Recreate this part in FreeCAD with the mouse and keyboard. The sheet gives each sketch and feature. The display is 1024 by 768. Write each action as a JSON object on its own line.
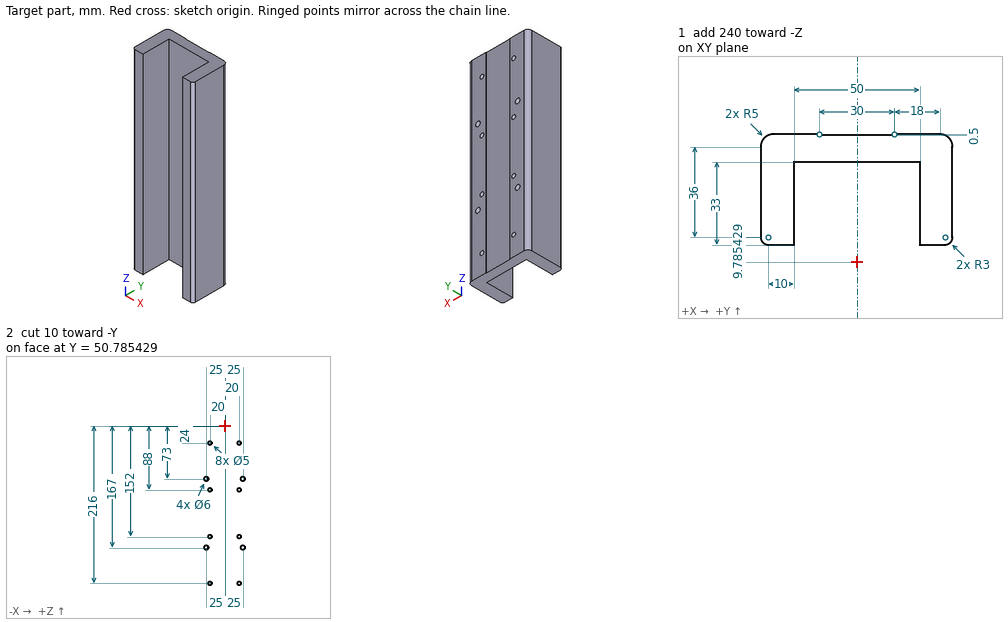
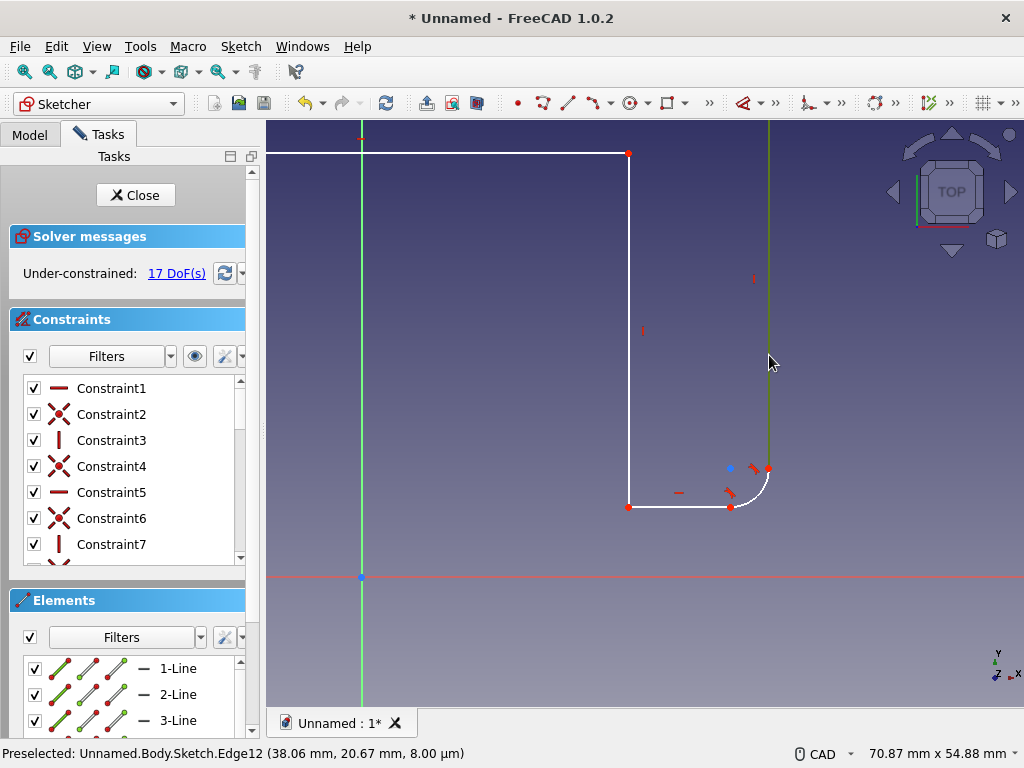
{"action": "scroll", "coordinate": [752, 502], "scroll_direction": "down", "scroll_amount": 4}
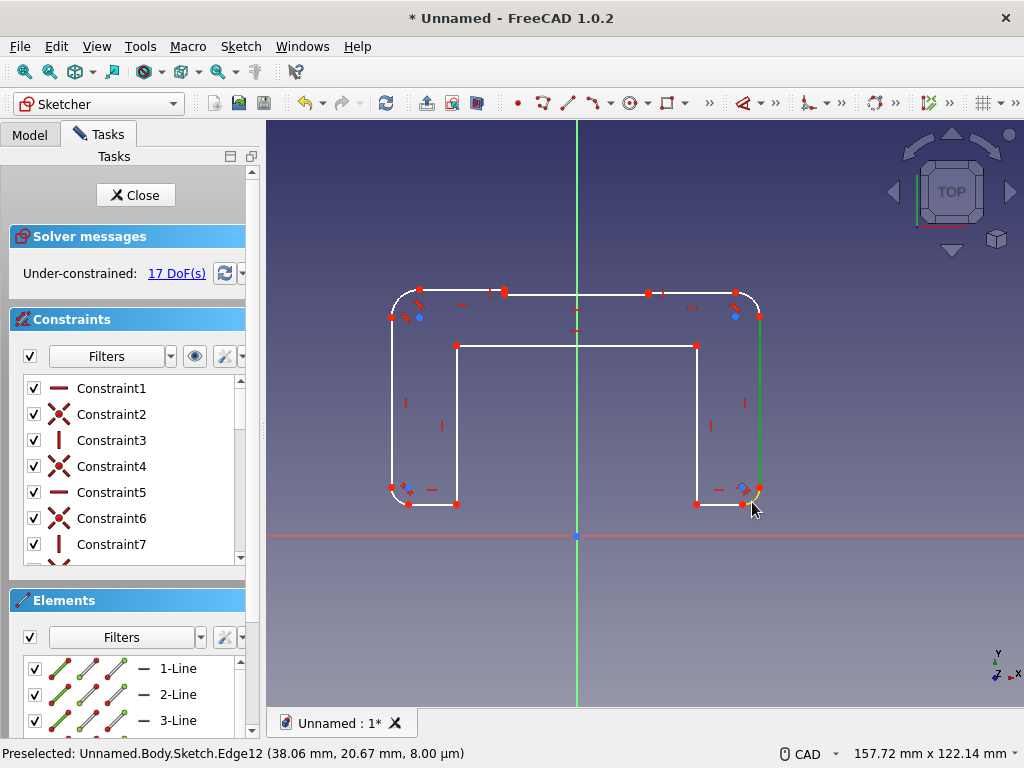
{"action": "scroll", "coordinate": [757, 306], "scroll_direction": "up", "scroll_amount": 2}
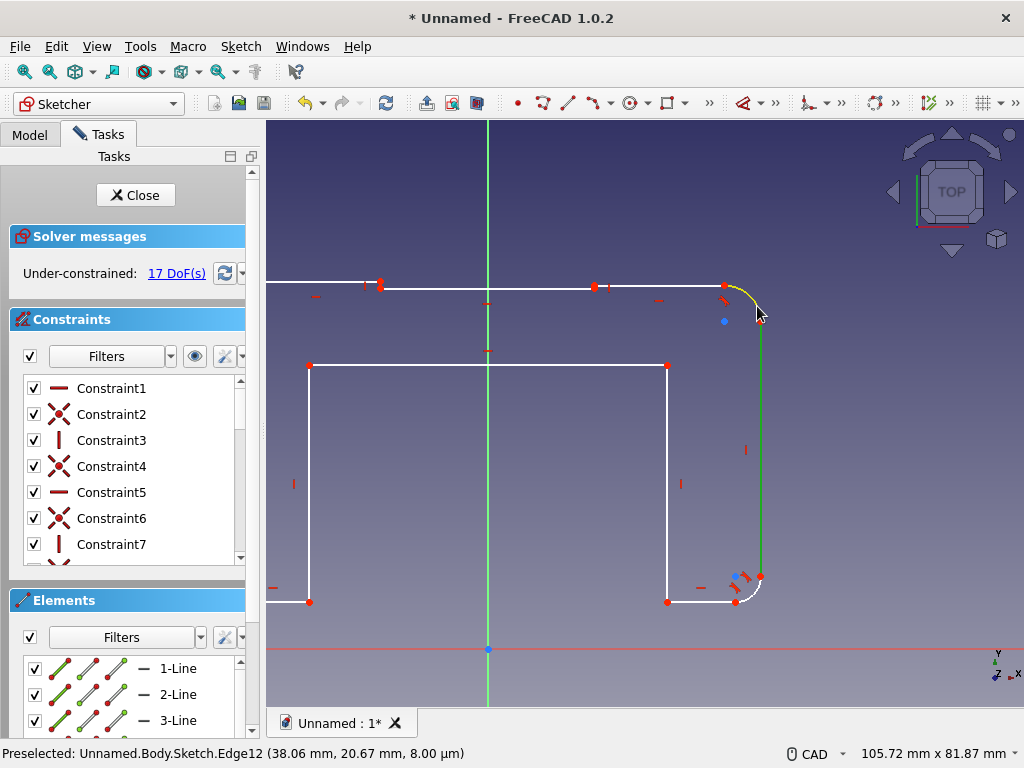
{"action": "left_click", "coordinate": [757, 305]}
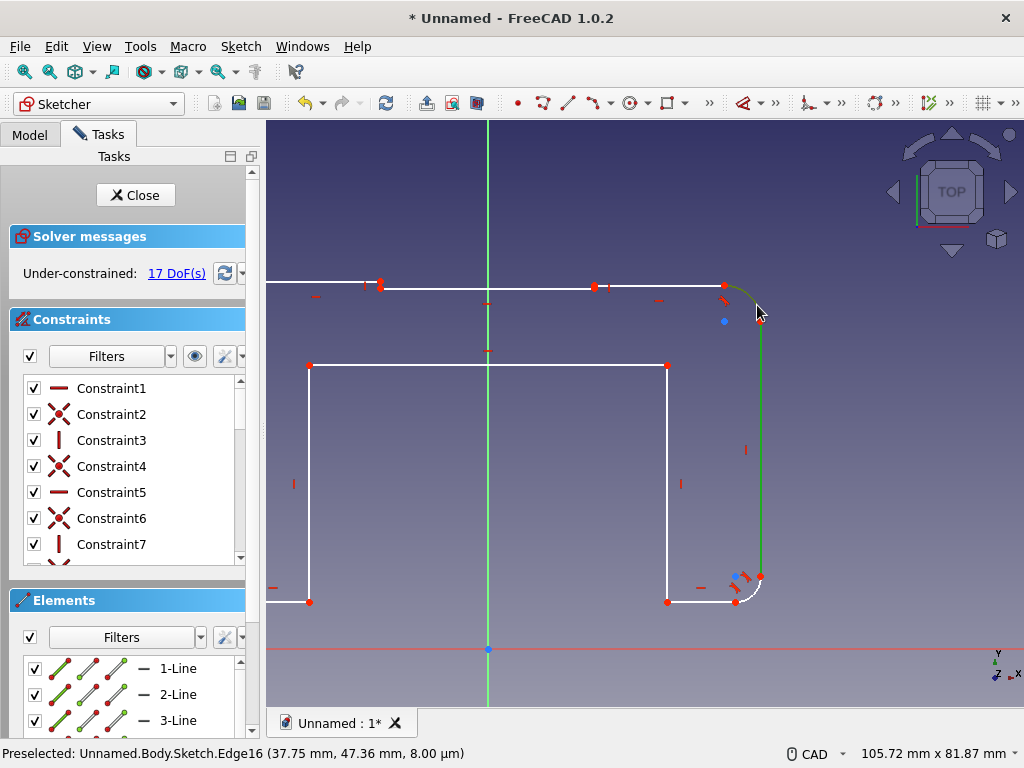
{"action": "key", "text": "t"}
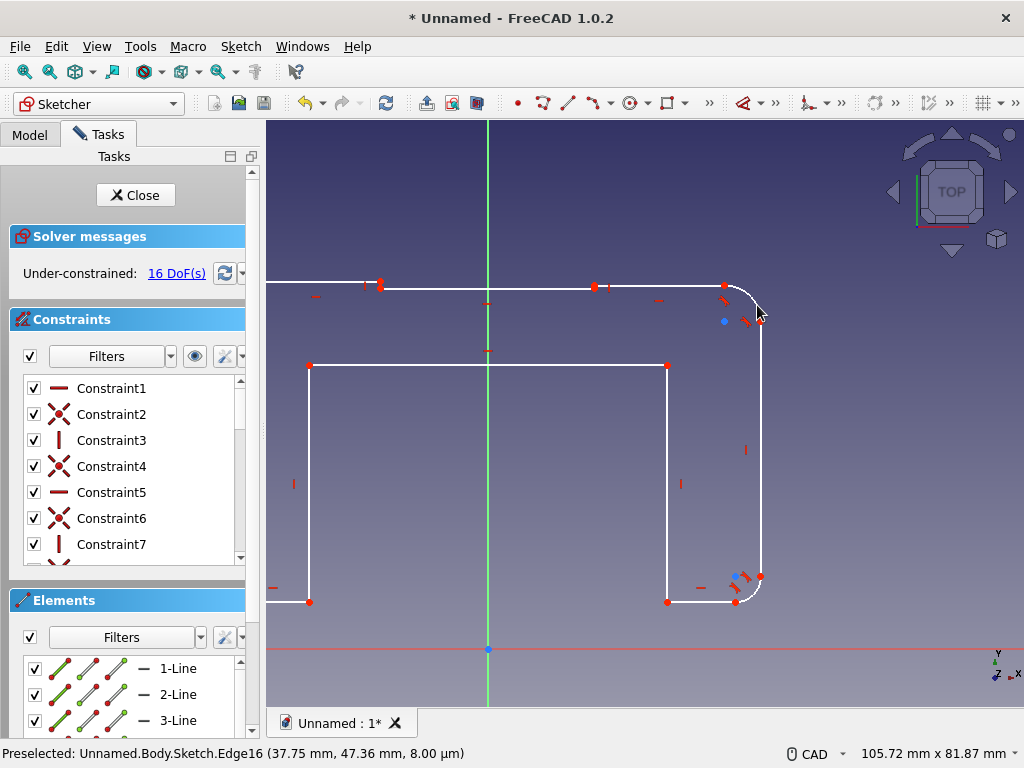
{"action": "scroll", "coordinate": [756, 305], "scroll_direction": "down", "scroll_amount": 2}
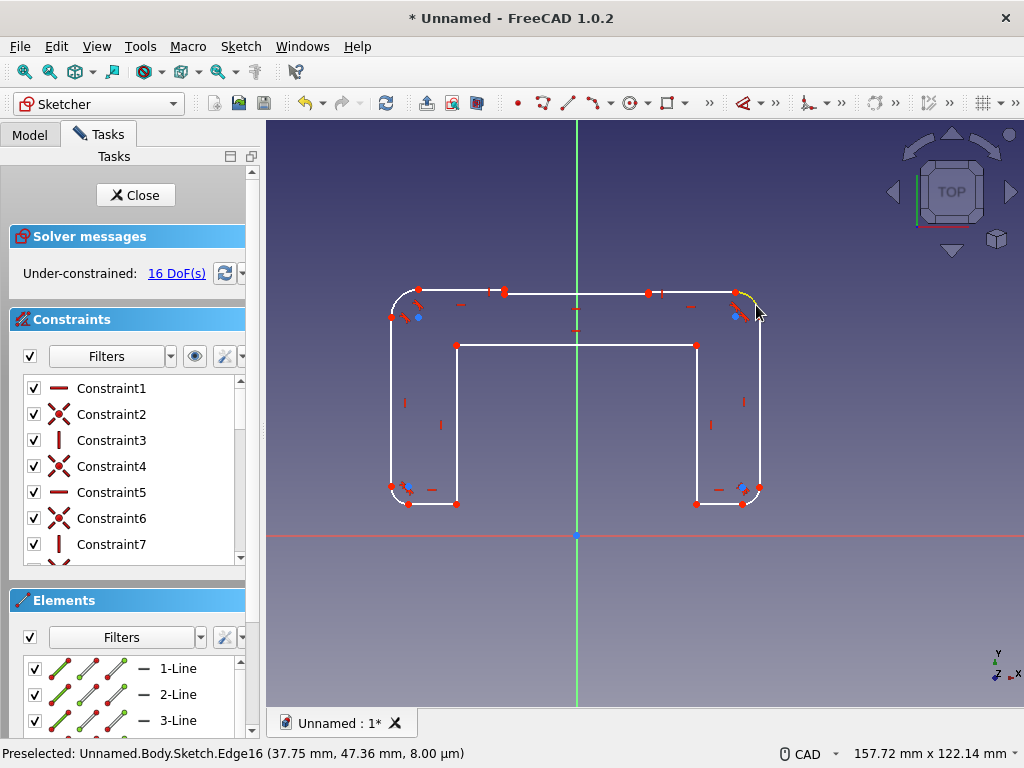
{"action": "scroll", "coordinate": [393, 495], "scroll_direction": "up", "scroll_amount": 3}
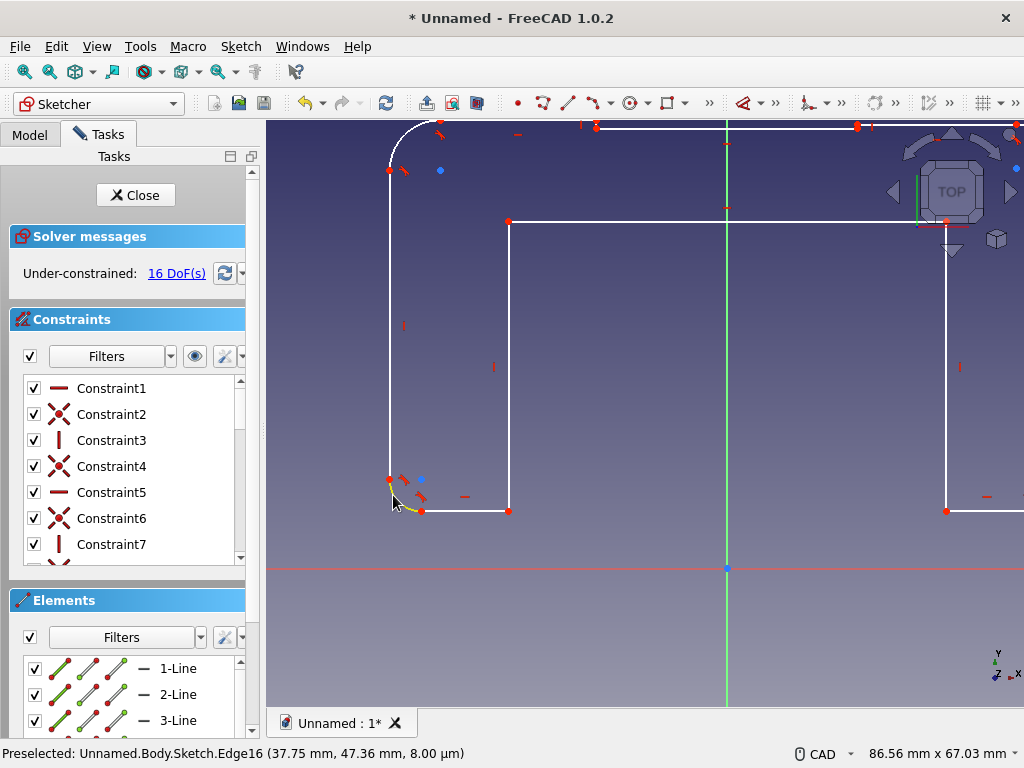
{"action": "left_click", "coordinate": [393, 494]}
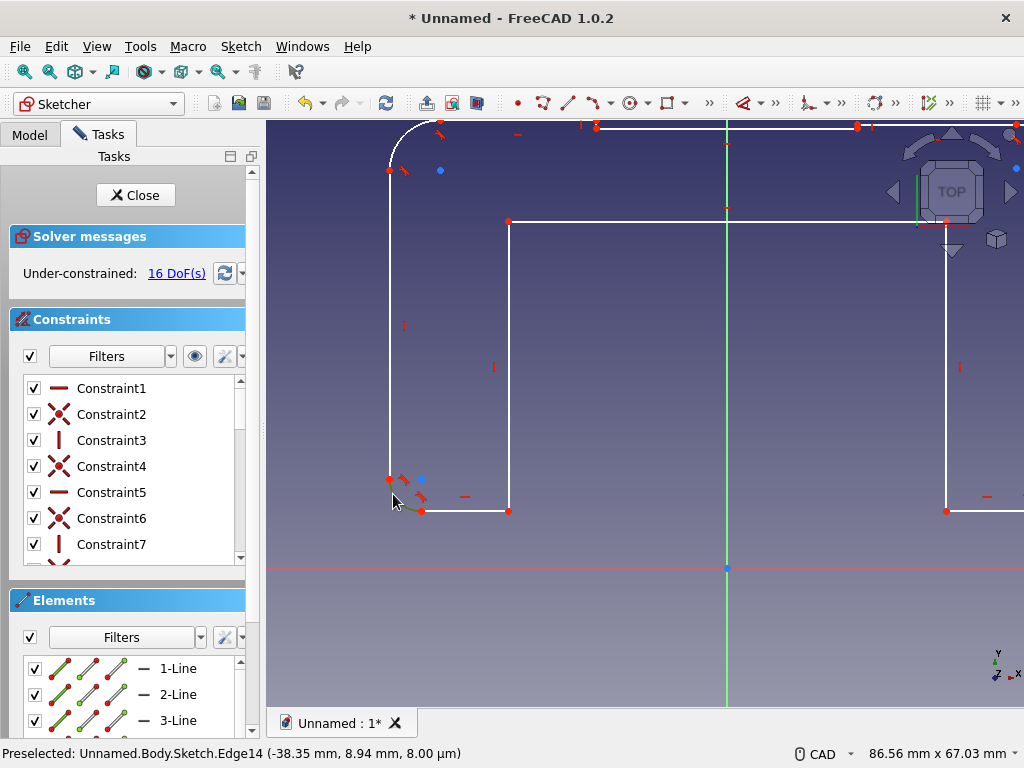
{"action": "scroll", "coordinate": [393, 495], "scroll_direction": "down", "scroll_amount": 3}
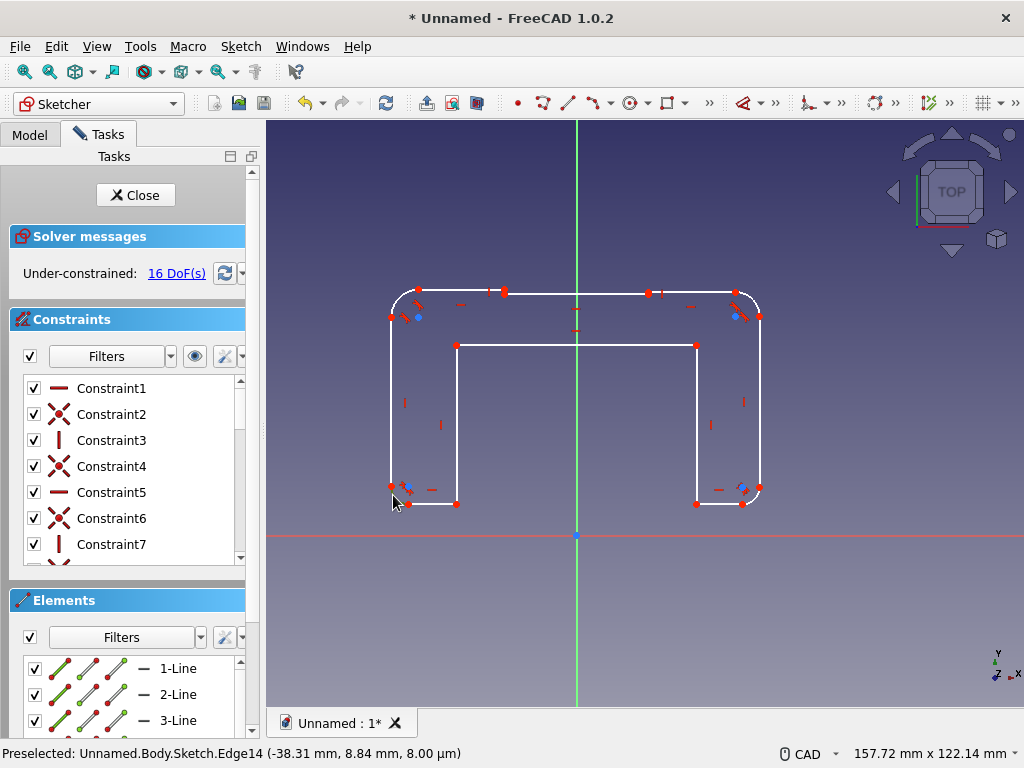
{"action": "scroll", "coordinate": [750, 502], "scroll_direction": "up", "scroll_amount": 3}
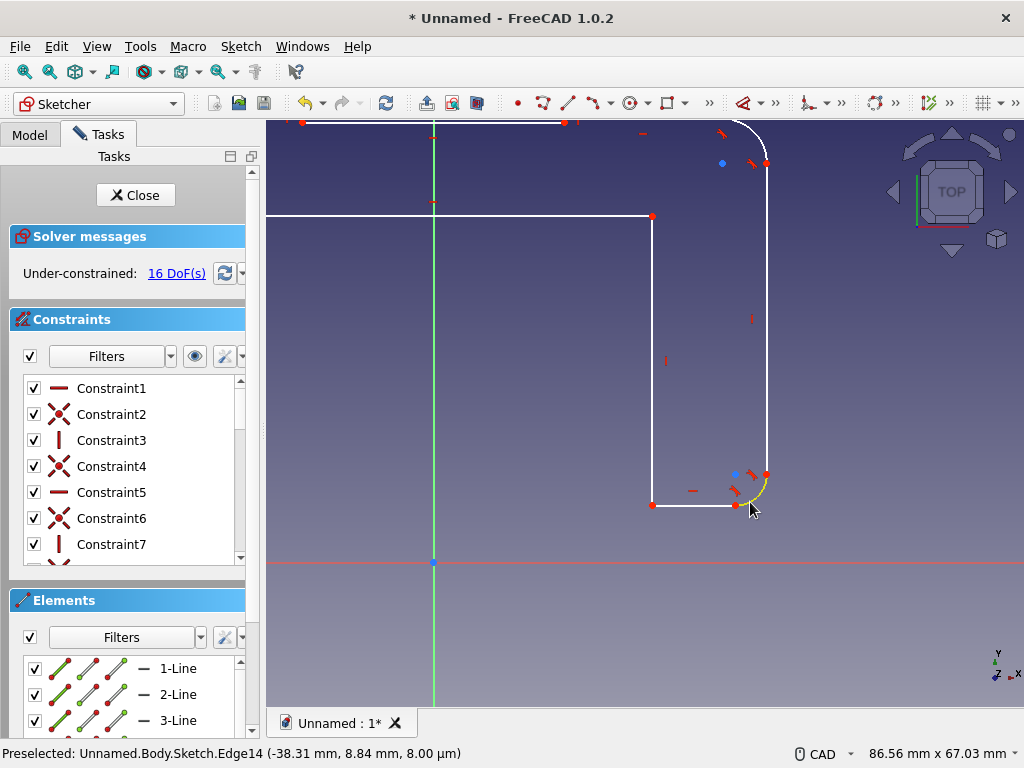
{"action": "left_click", "coordinate": [750, 502]}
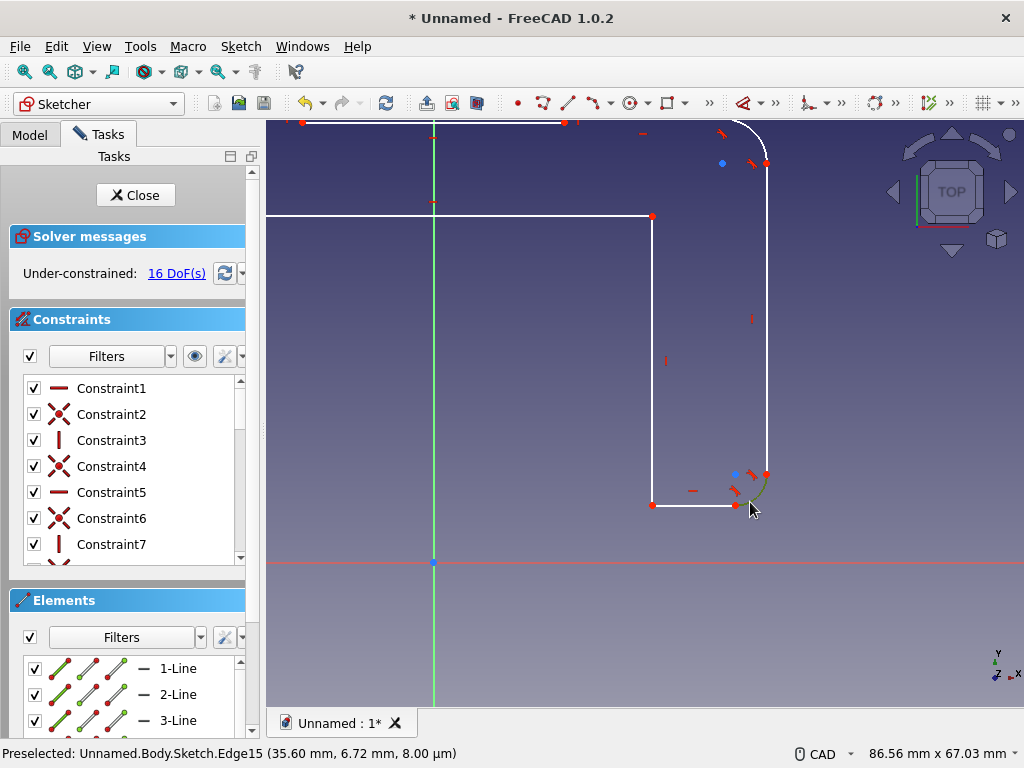
{"action": "key", "text": "e"}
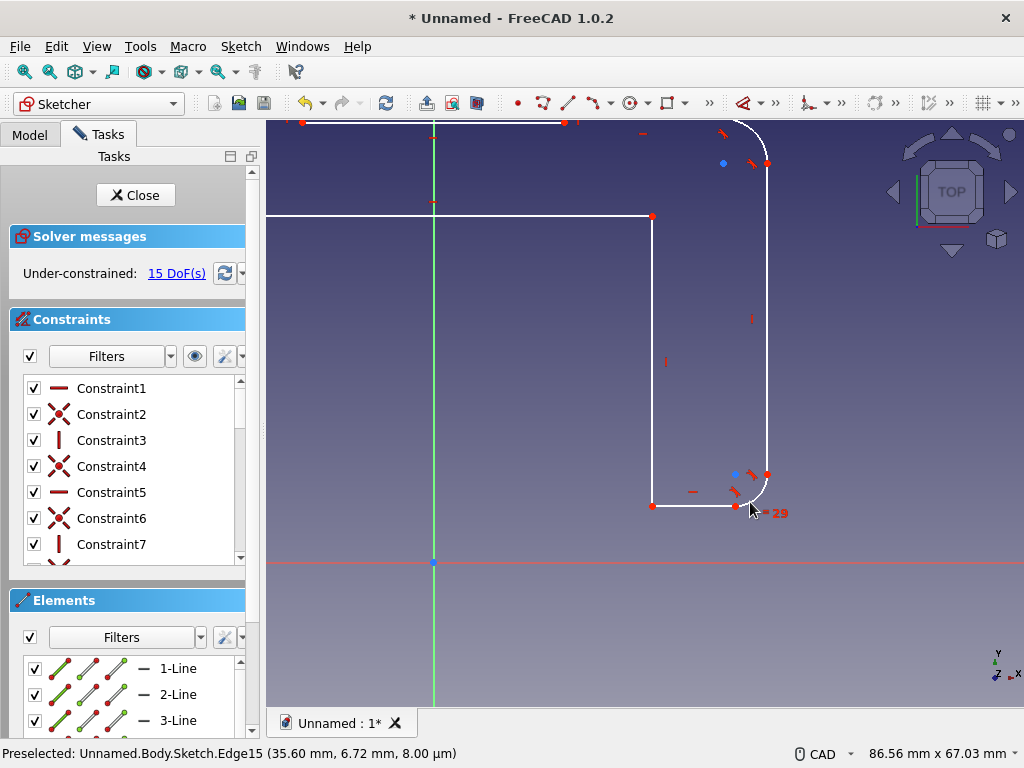
{"action": "scroll", "coordinate": [750, 502], "scroll_direction": "down", "scroll_amount": 3}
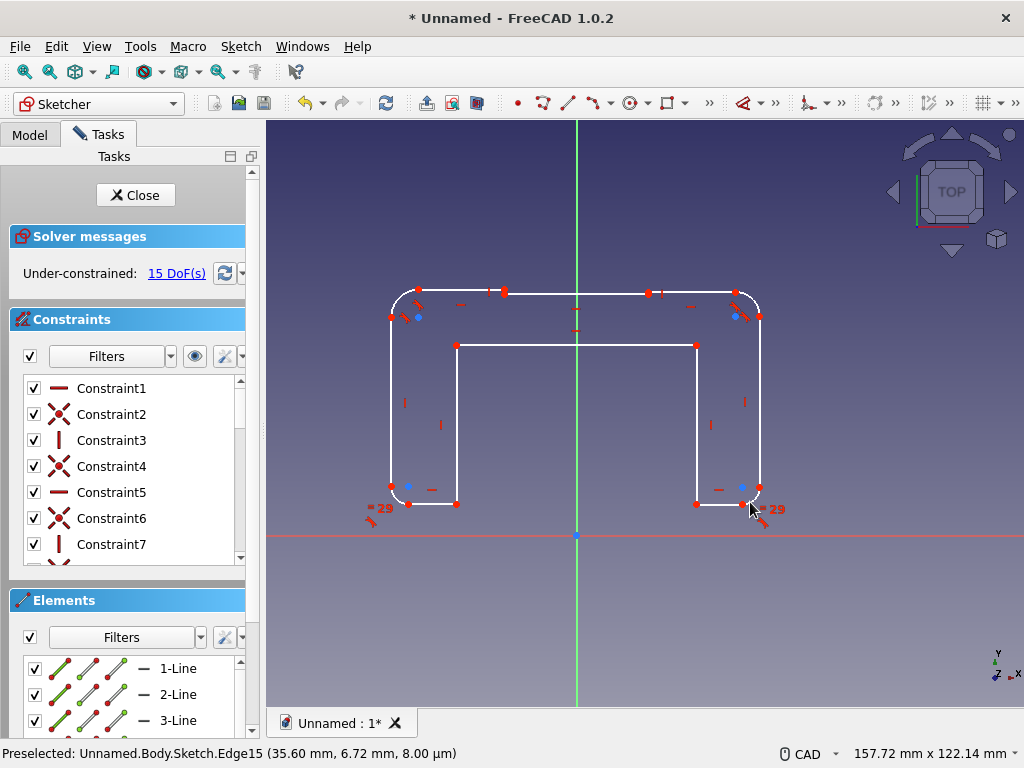
{"action": "left_click", "coordinate": [406, 293]}